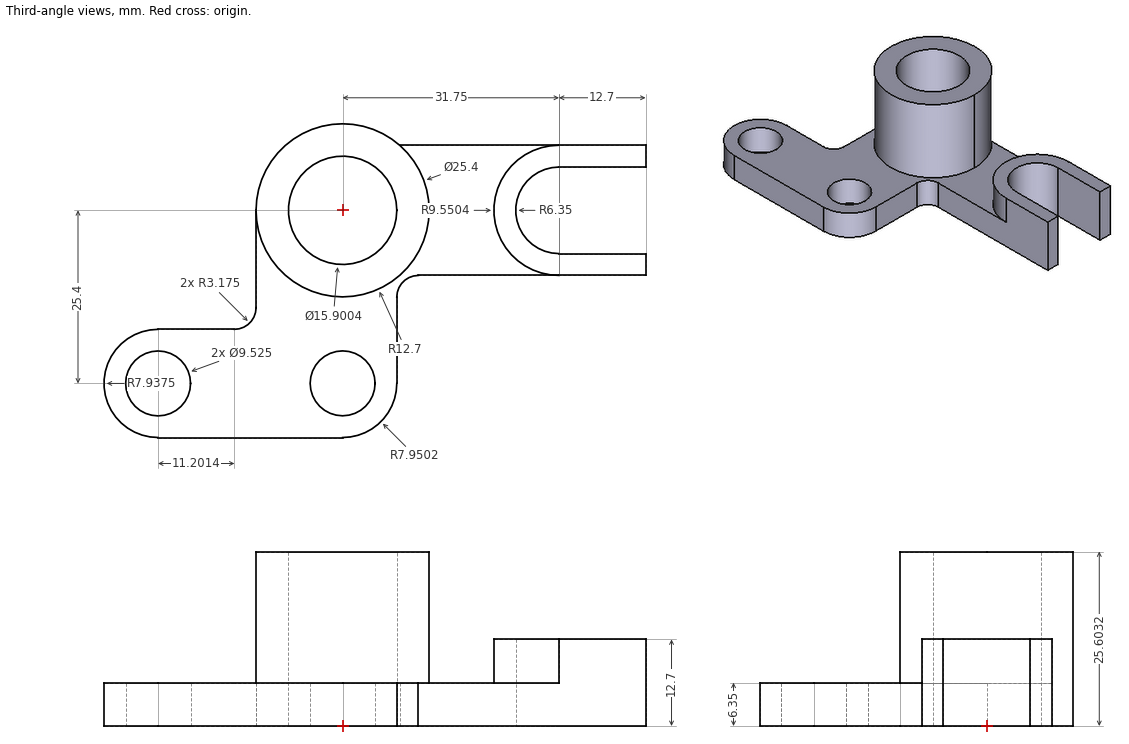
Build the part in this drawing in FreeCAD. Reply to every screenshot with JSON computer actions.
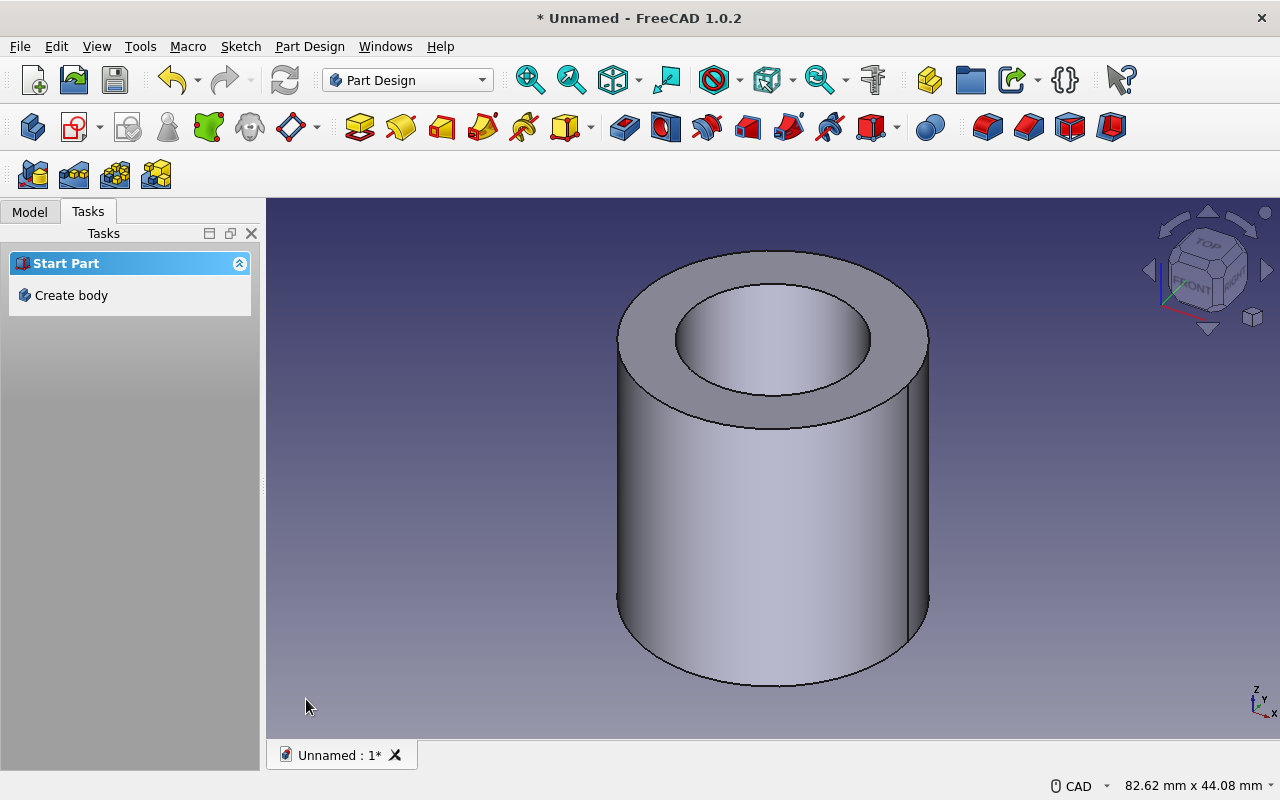
{"action": "left_click", "coordinate": [74, 128]}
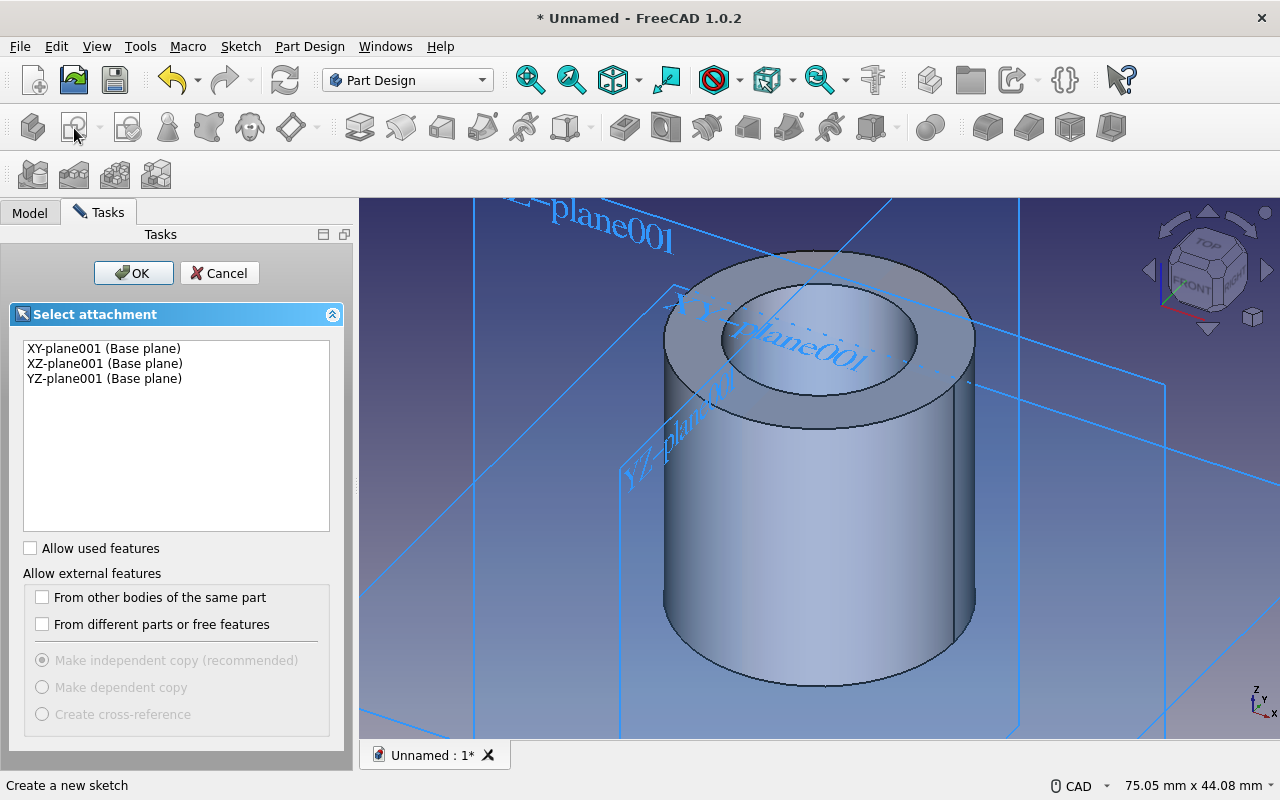
{"action": "left_click", "coordinate": [84, 348]}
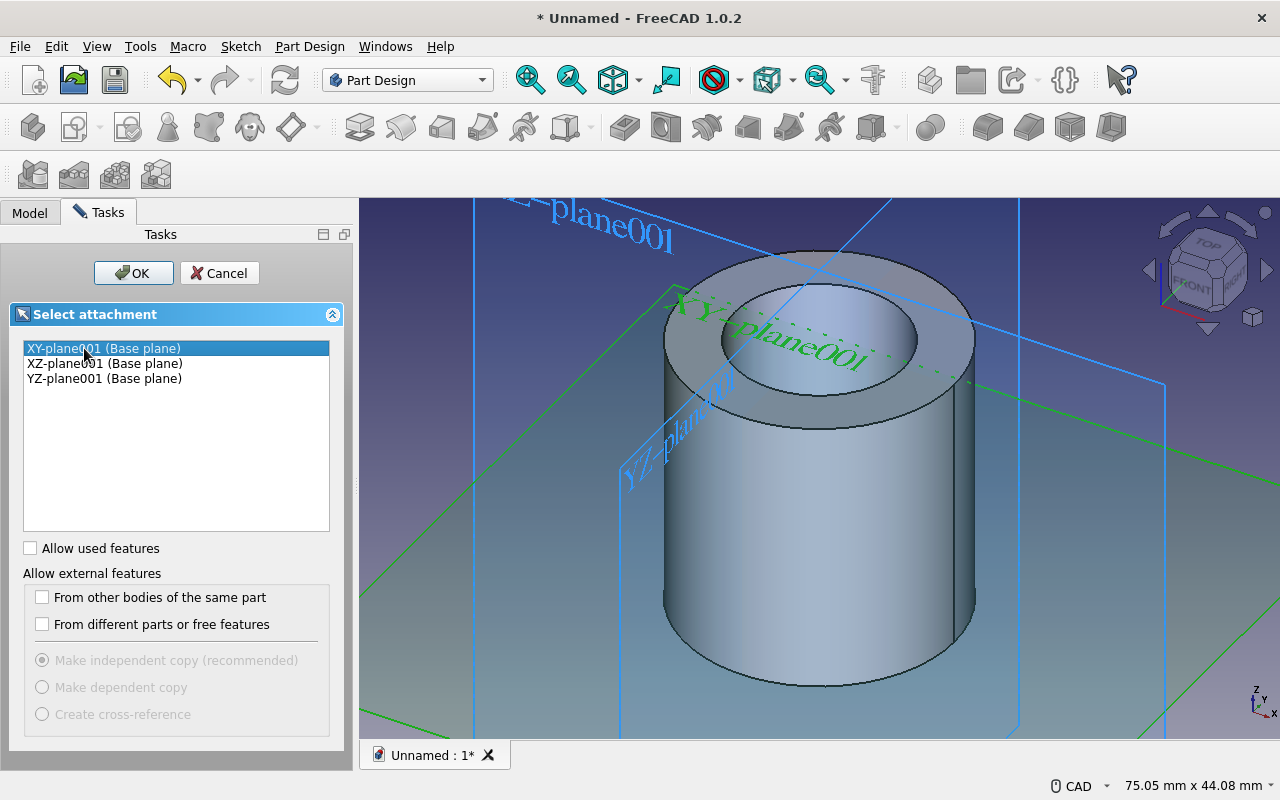
{"action": "left_click", "coordinate": [134, 273]}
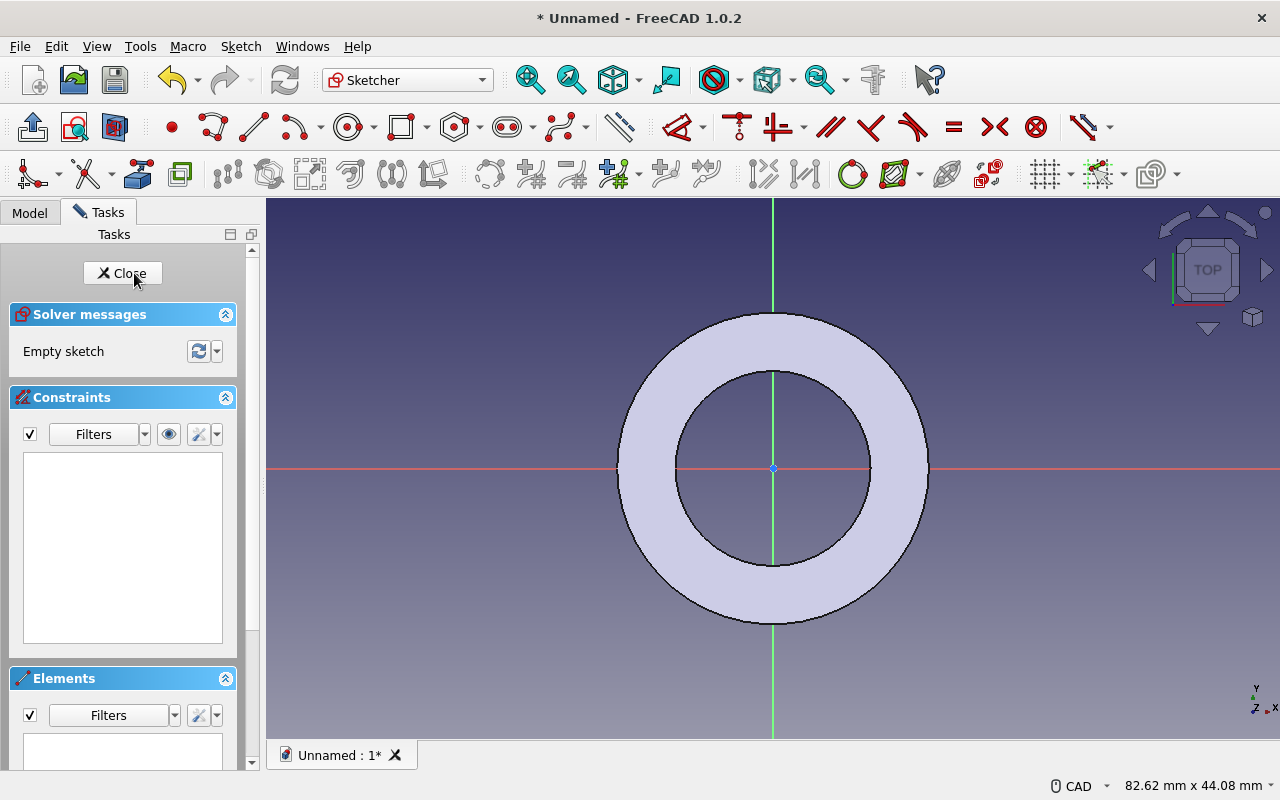
{"action": "scroll", "coordinate": [294, 468], "scroll_direction": "down", "scroll_amount": 2}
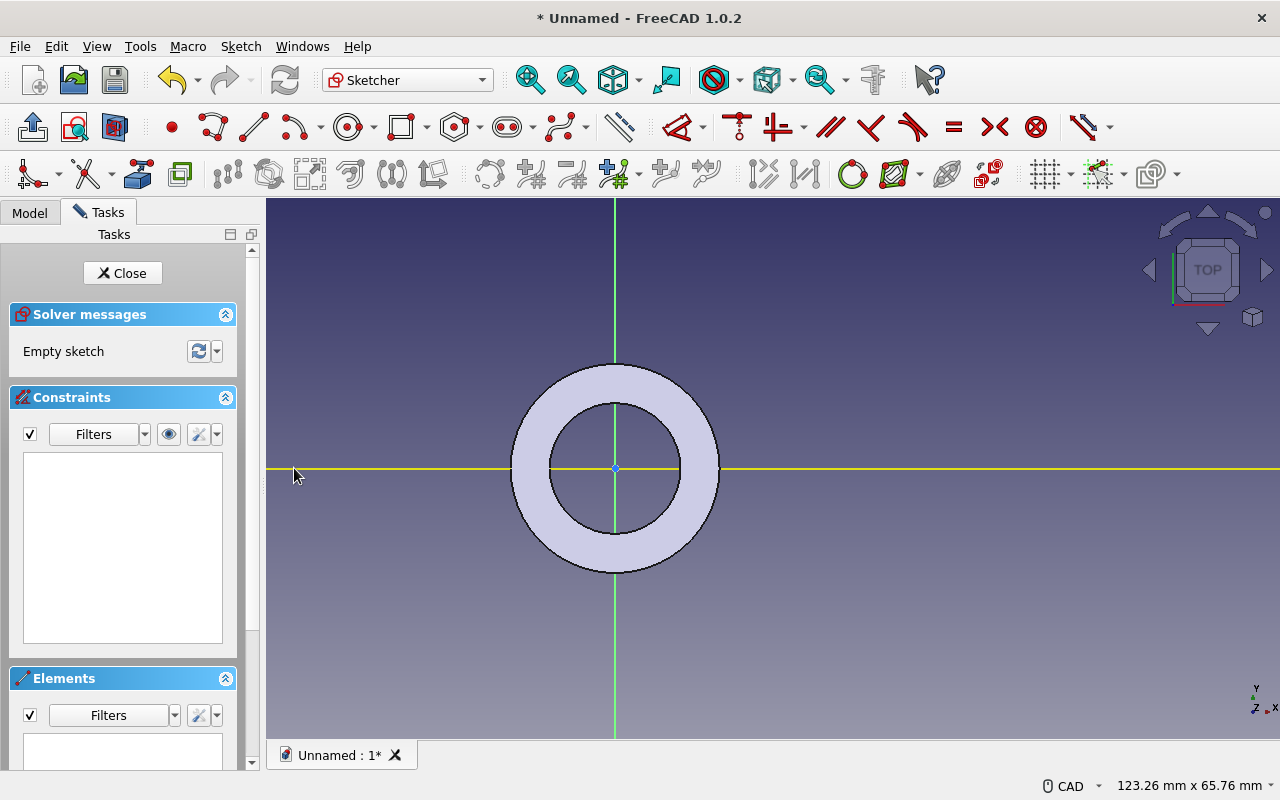
{"action": "scroll", "coordinate": [988, 469], "scroll_direction": "up", "scroll_amount": 2}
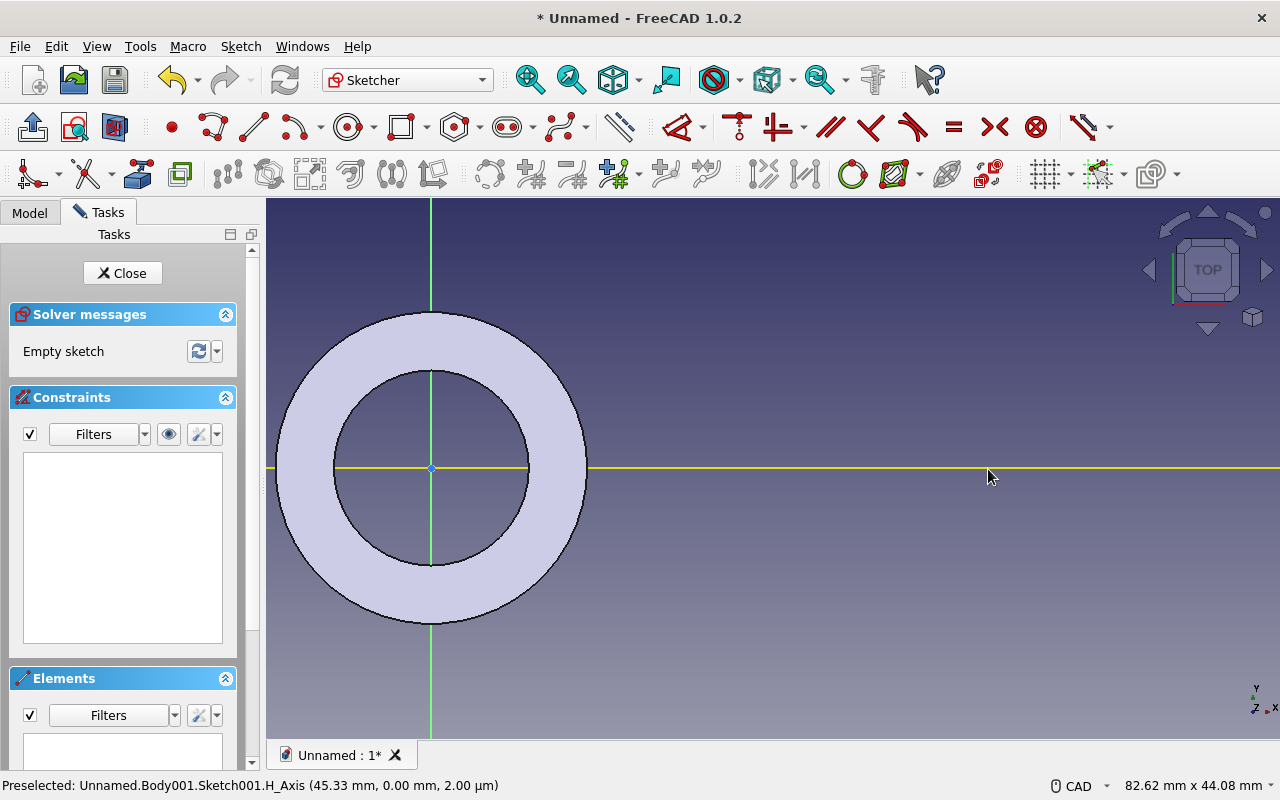
{"action": "left_click", "coordinate": [213, 128]}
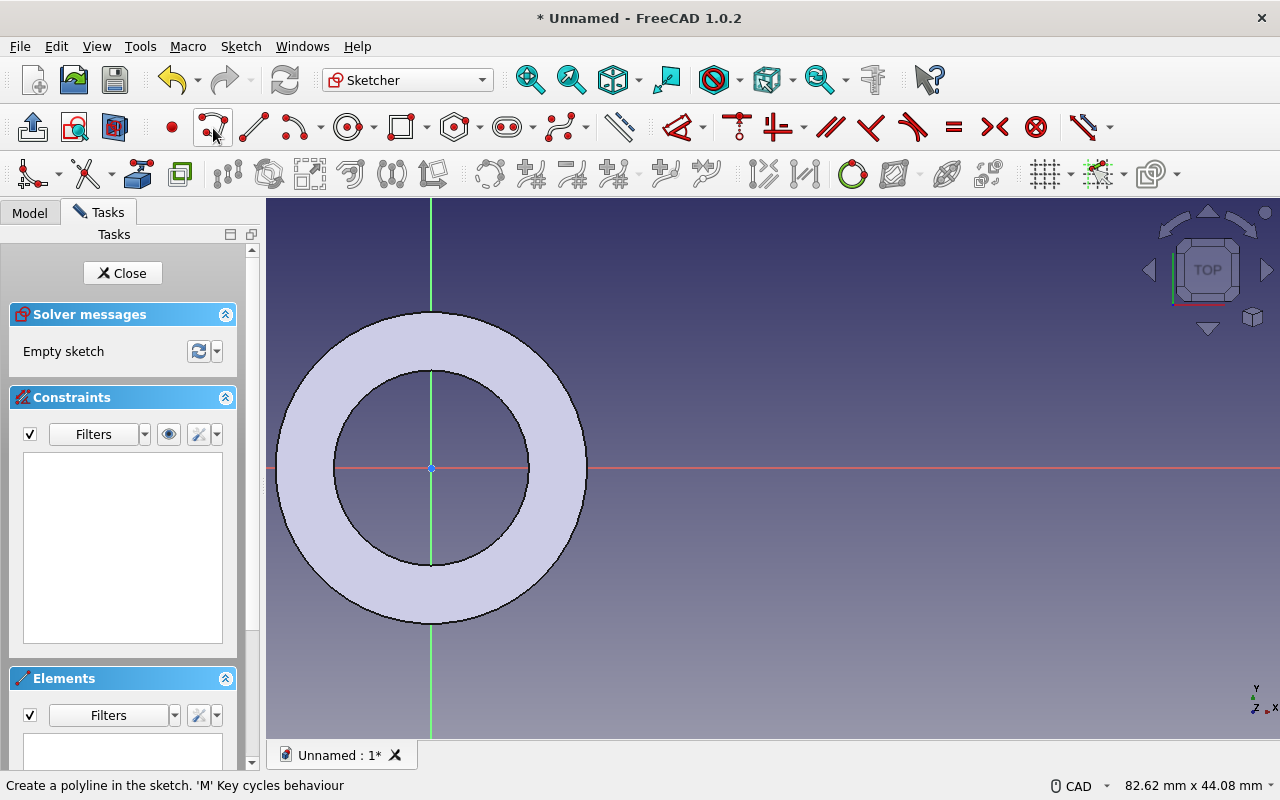
{"action": "left_click", "coordinate": [821, 585]}
{"action": "left_click", "coordinate": [977, 585]}
{"action": "left_click", "coordinate": [977, 546]}
{"action": "left_click", "coordinate": [821, 546]}
{"action": "right_click", "coordinate": [821, 546]}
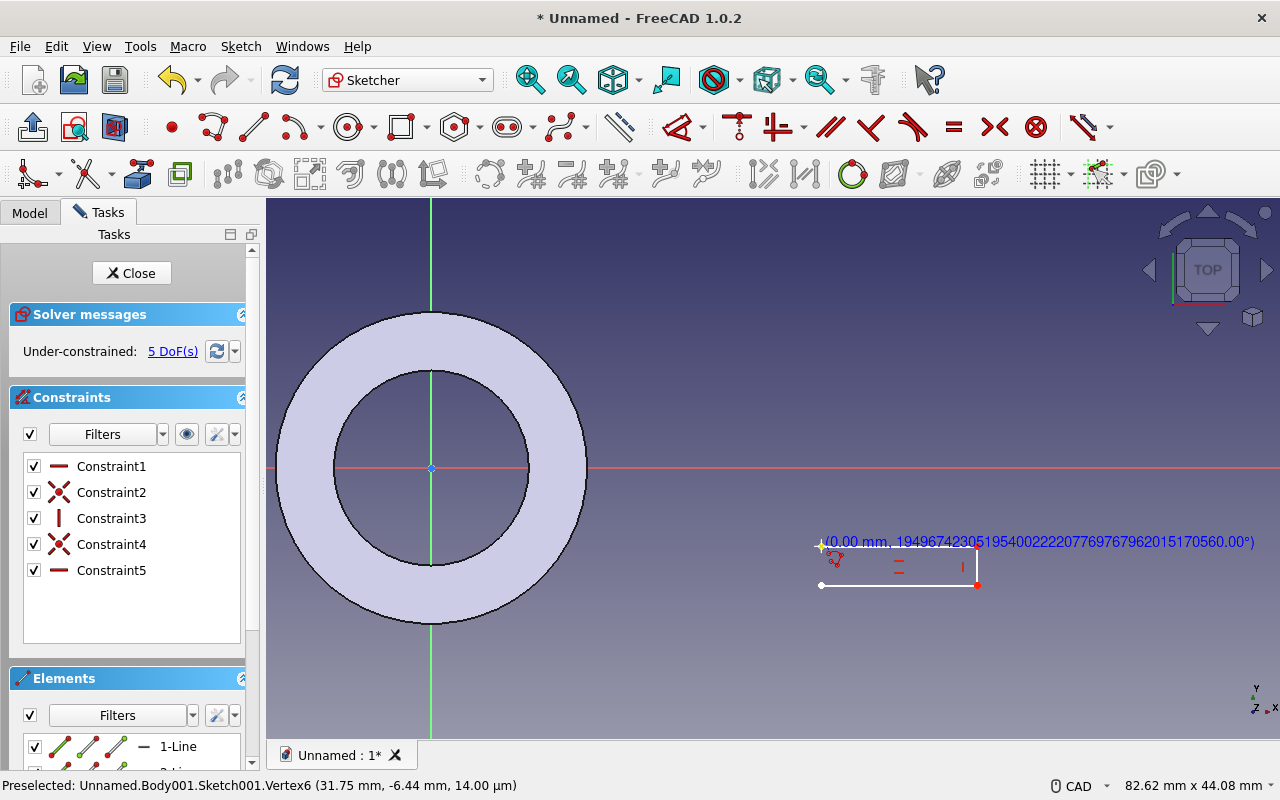
{"action": "left_click", "coordinate": [821, 390]}
{"action": "left_click", "coordinate": [977, 390]}
{"action": "left_click", "coordinate": [977, 351]}
{"action": "left_click", "coordinate": [821, 351]}
{"action": "right_click", "coordinate": [821, 351]}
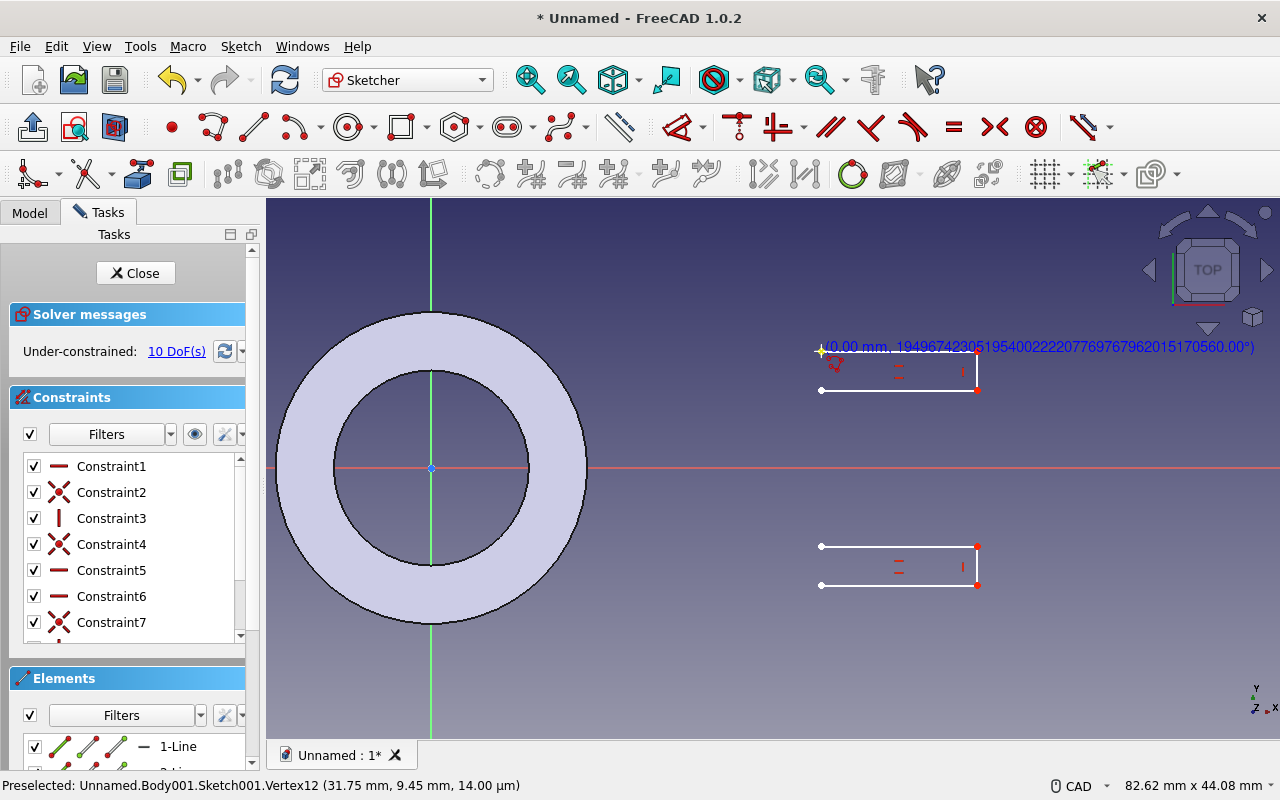
{"action": "left_click", "coordinate": [320, 128]}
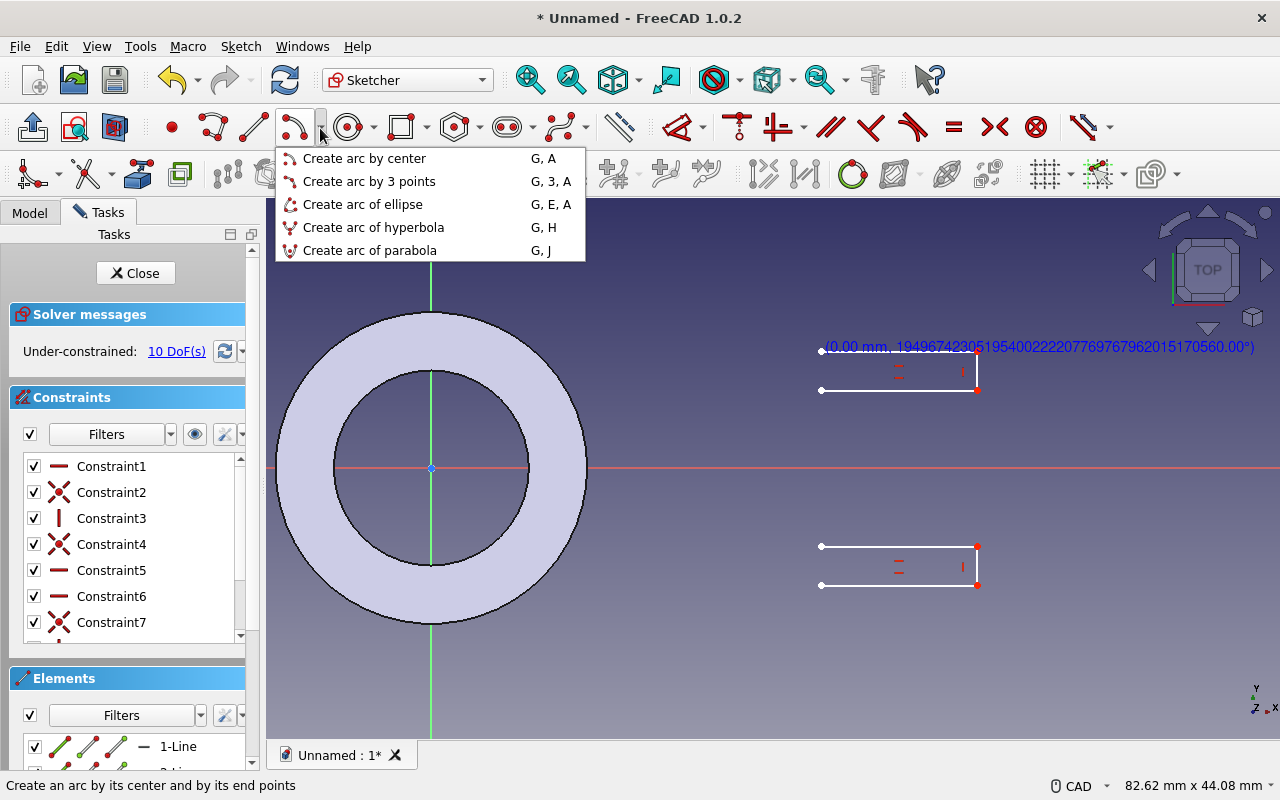
{"action": "left_click", "coordinate": [430, 182]}